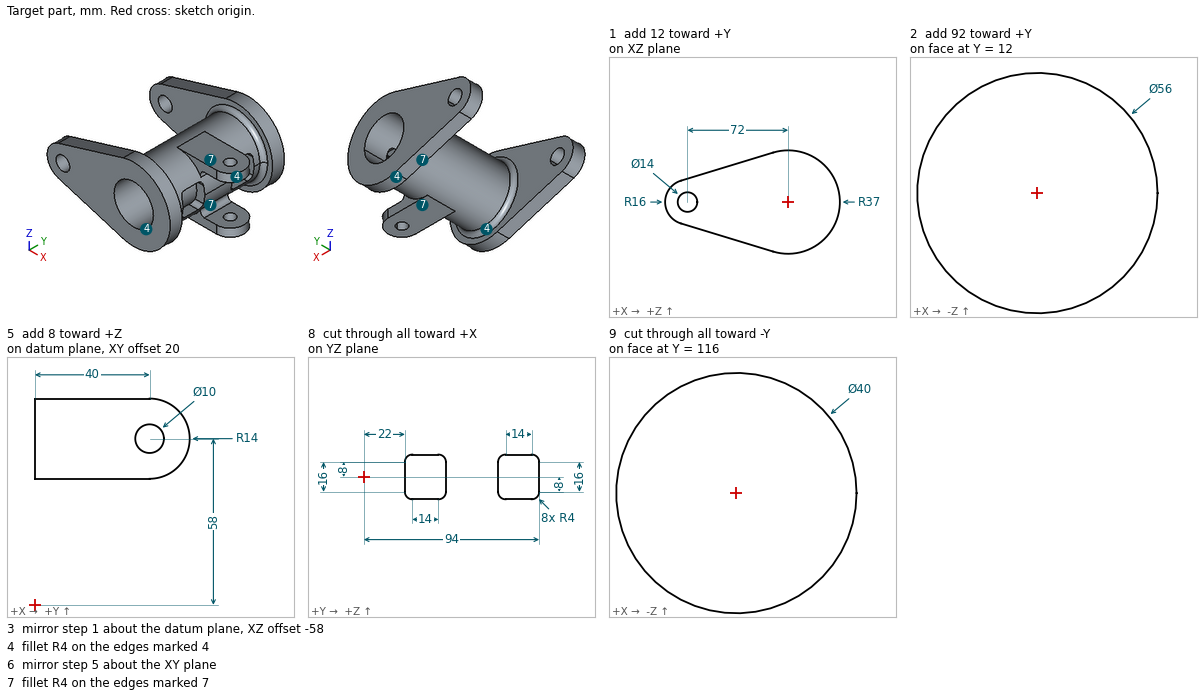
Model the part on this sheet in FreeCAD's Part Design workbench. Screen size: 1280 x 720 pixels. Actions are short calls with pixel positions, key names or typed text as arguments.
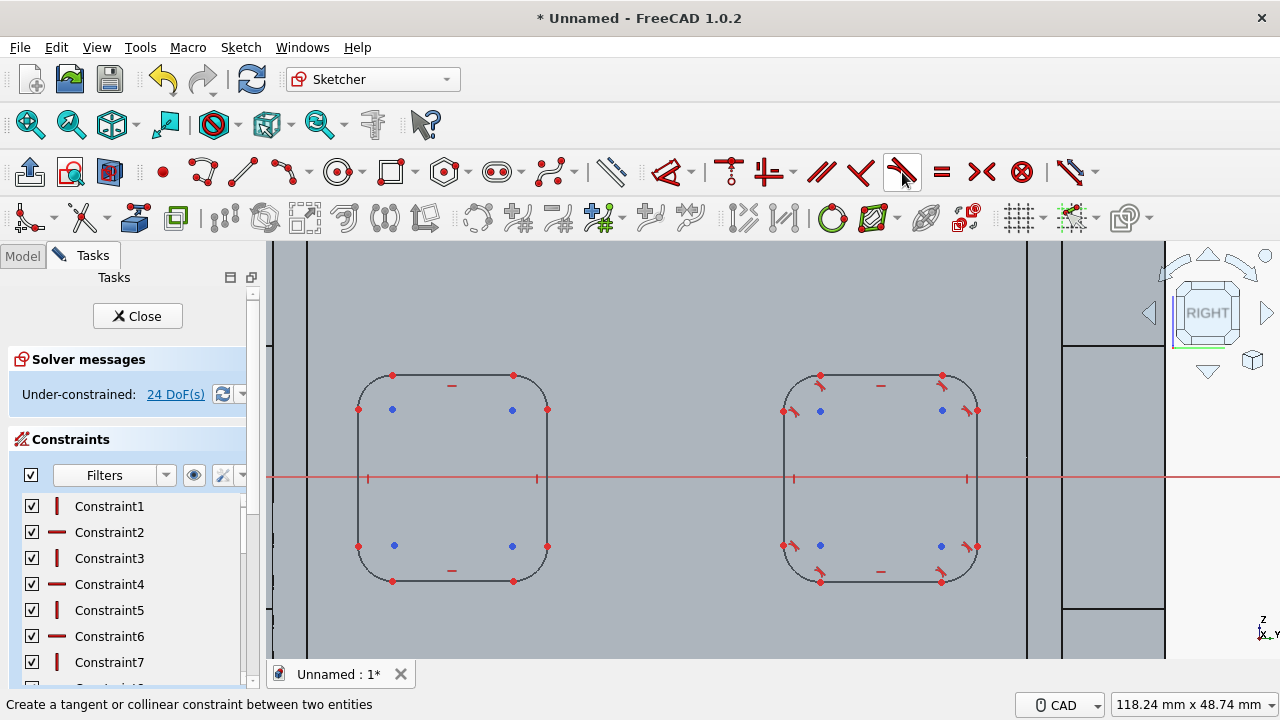
click(358, 451)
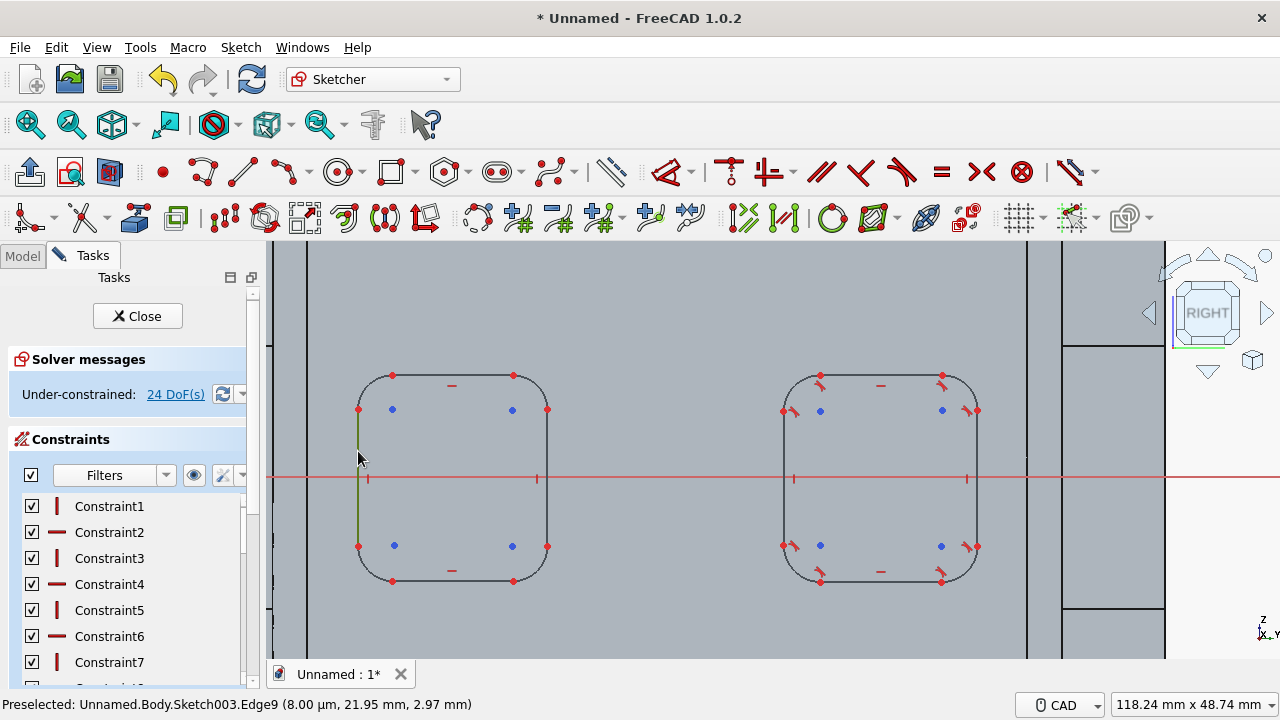
click(362, 562)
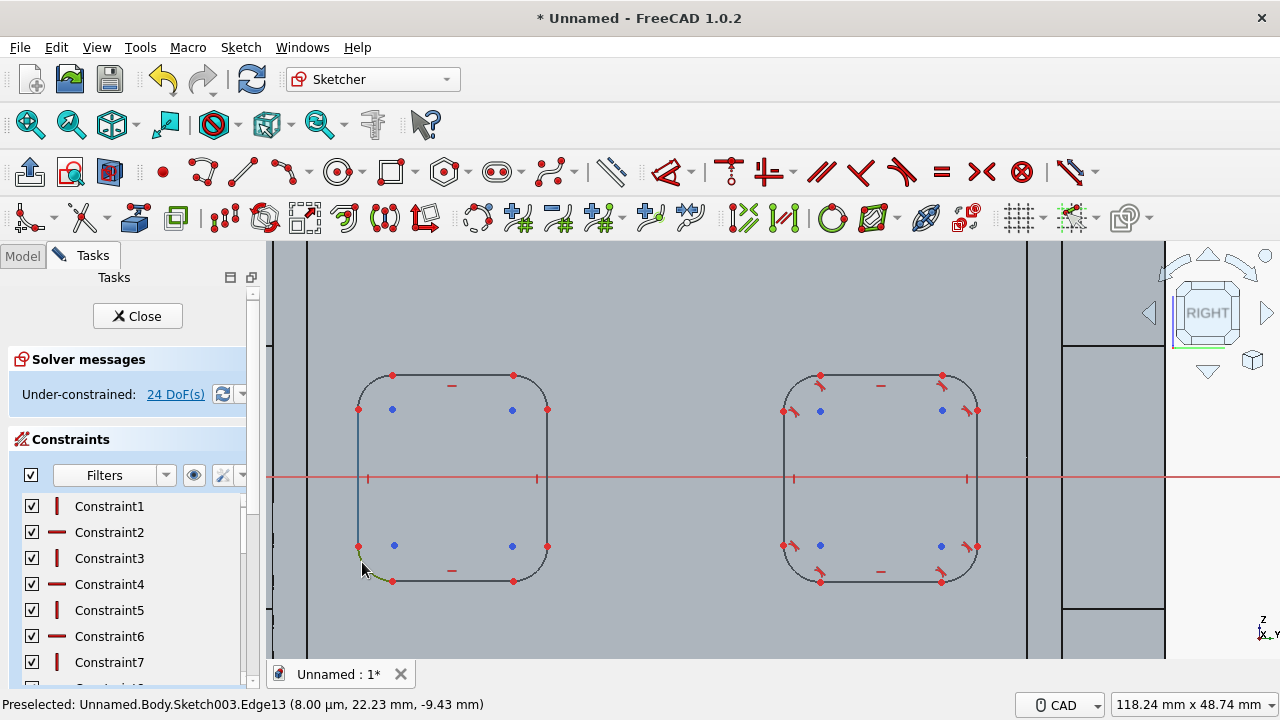
key(t)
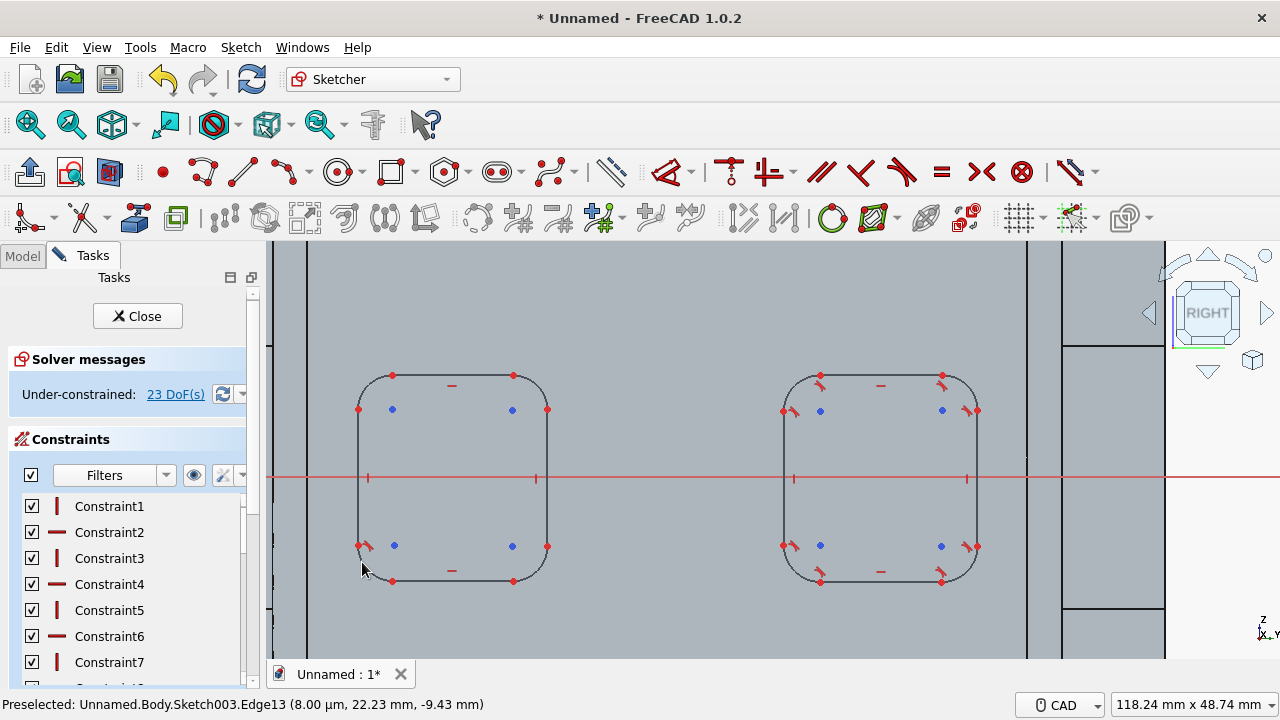
click(358, 450)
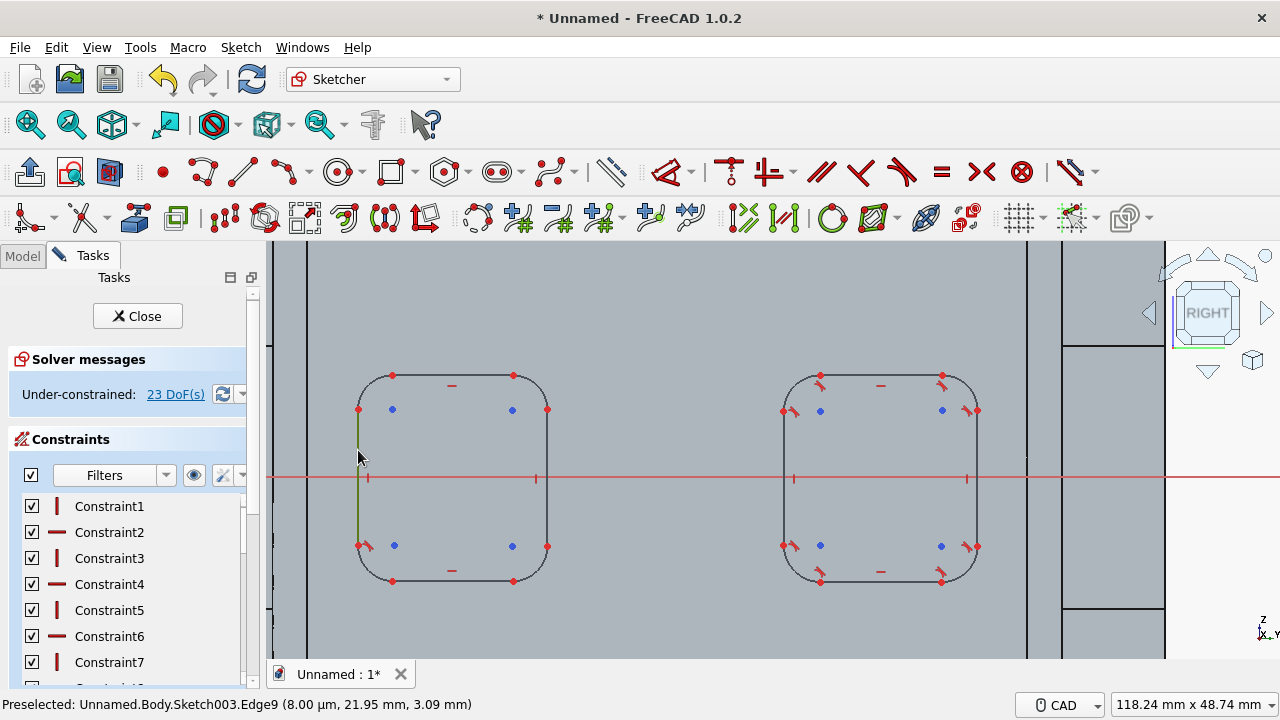
click(377, 379)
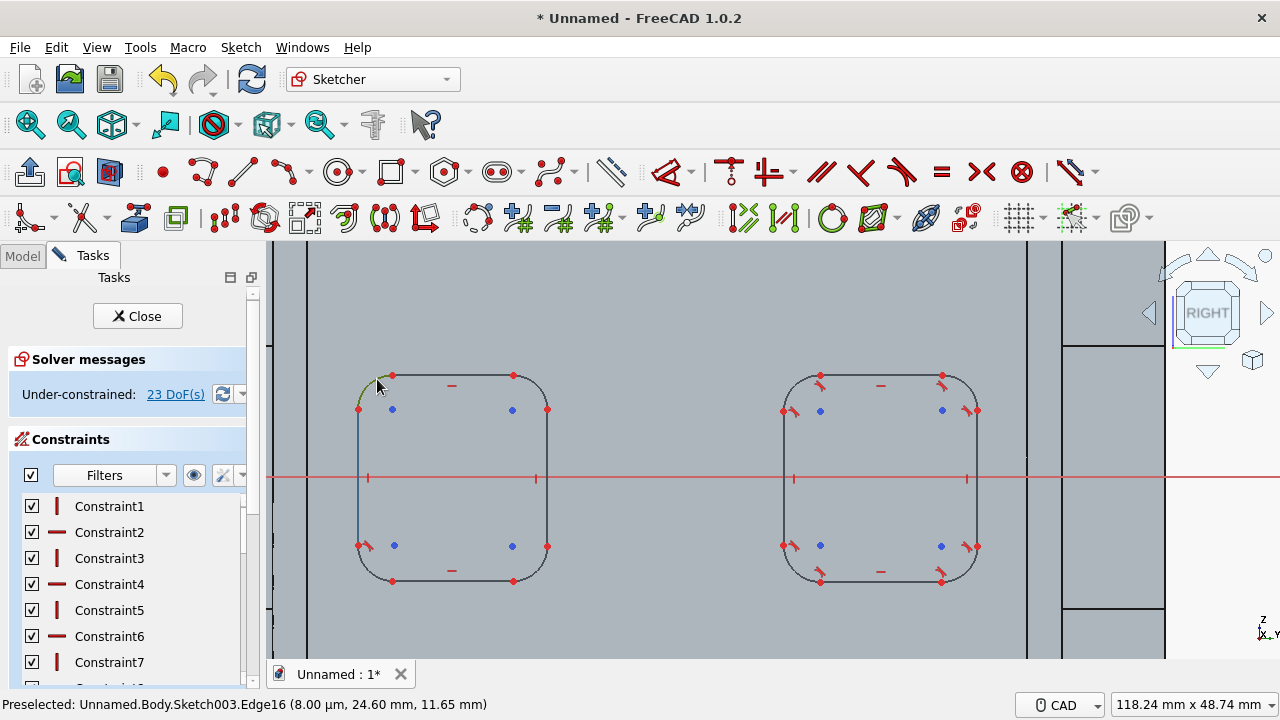
click(902, 172)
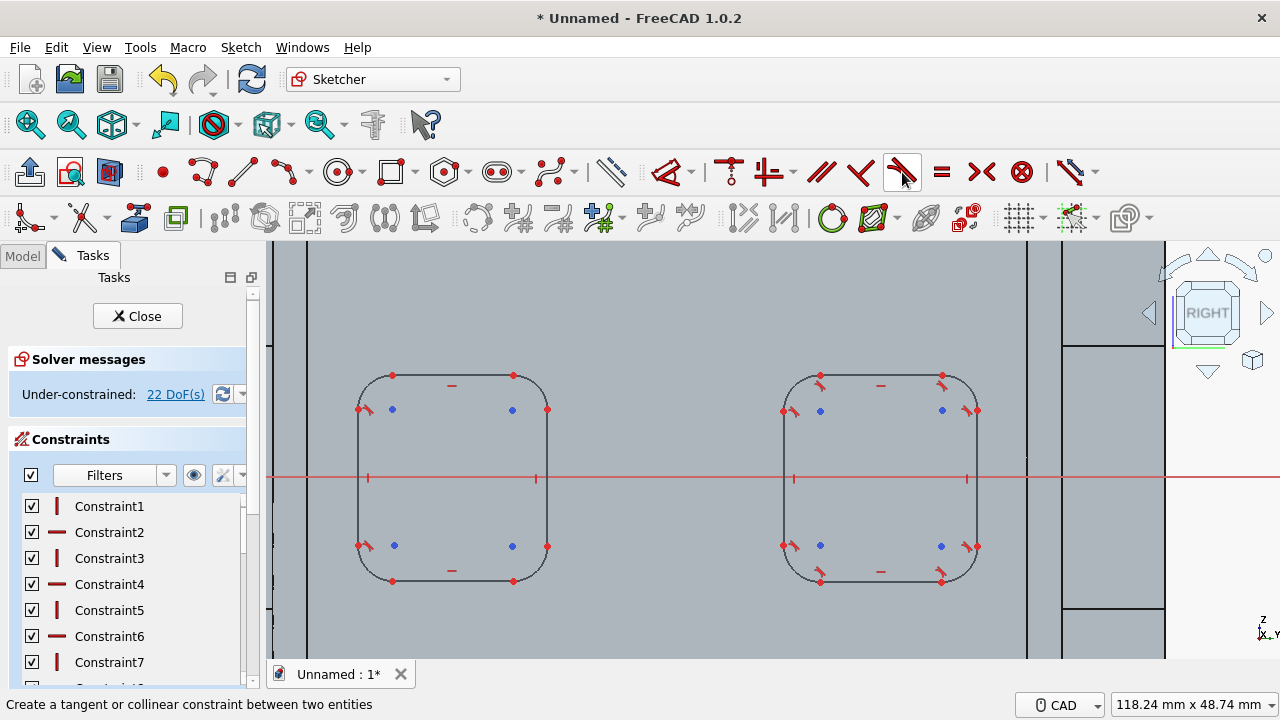
click(429, 581)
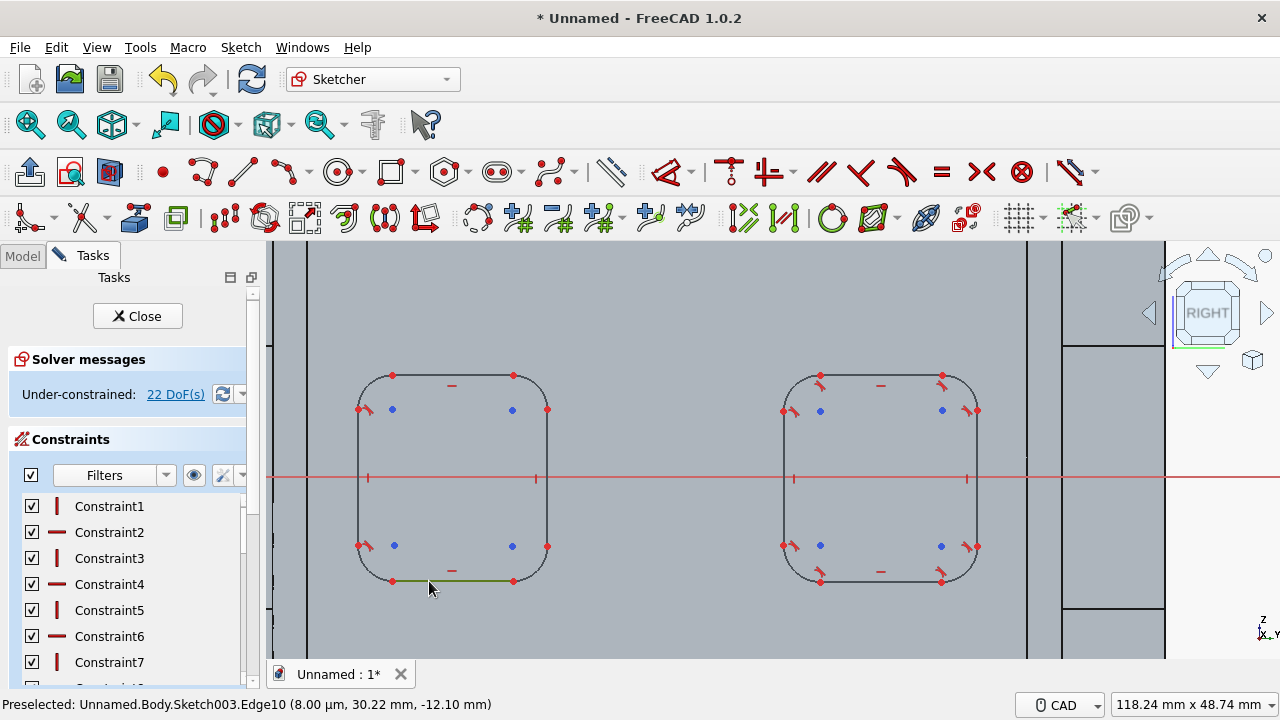
click(362, 561)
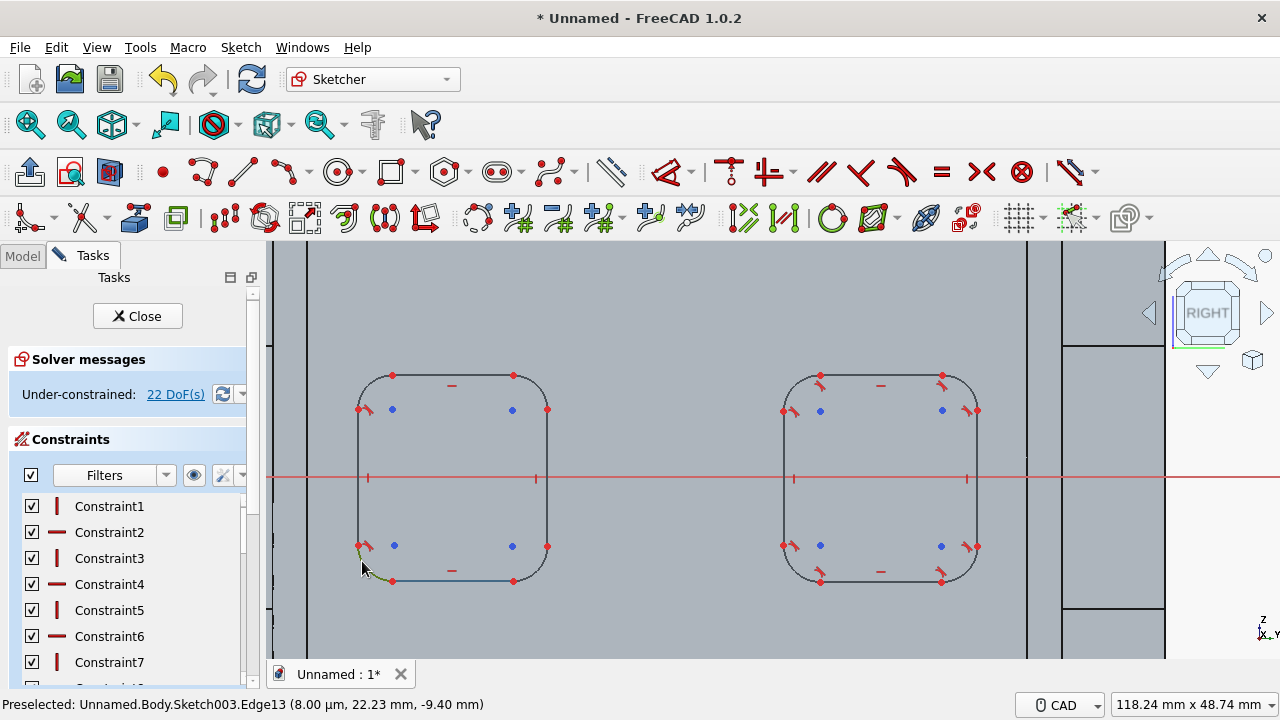
click(902, 172)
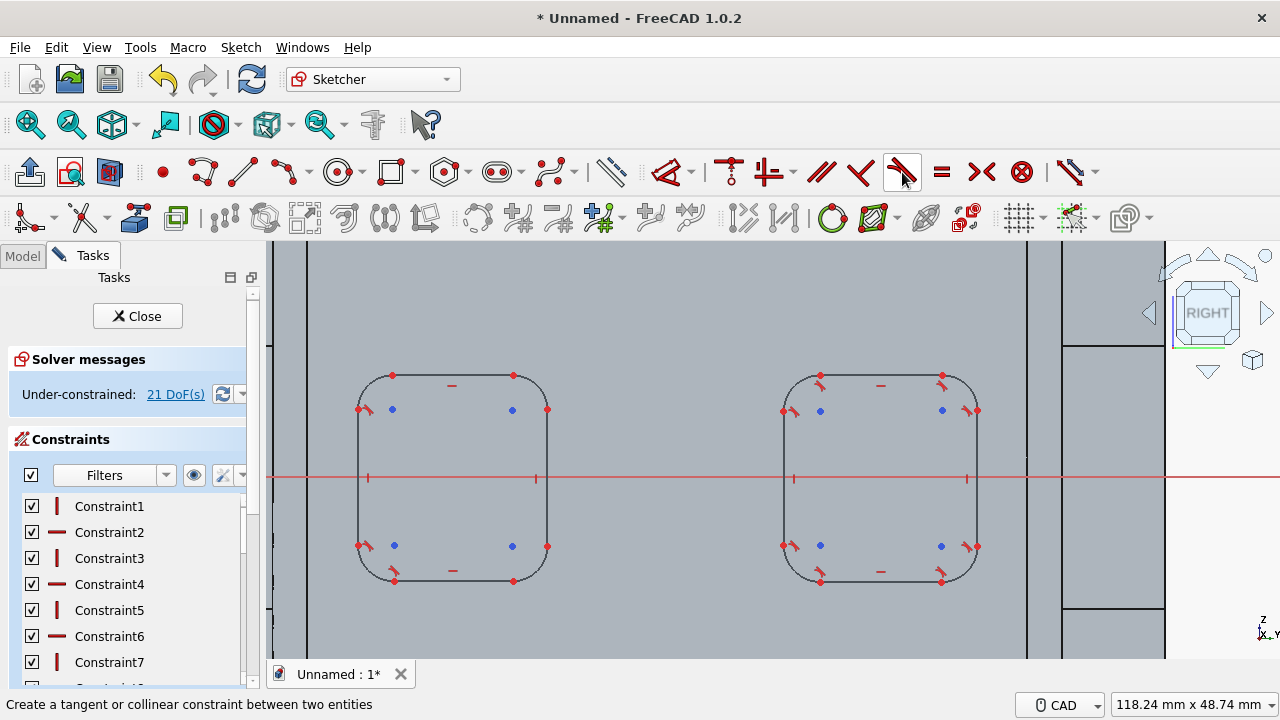
click(430, 581)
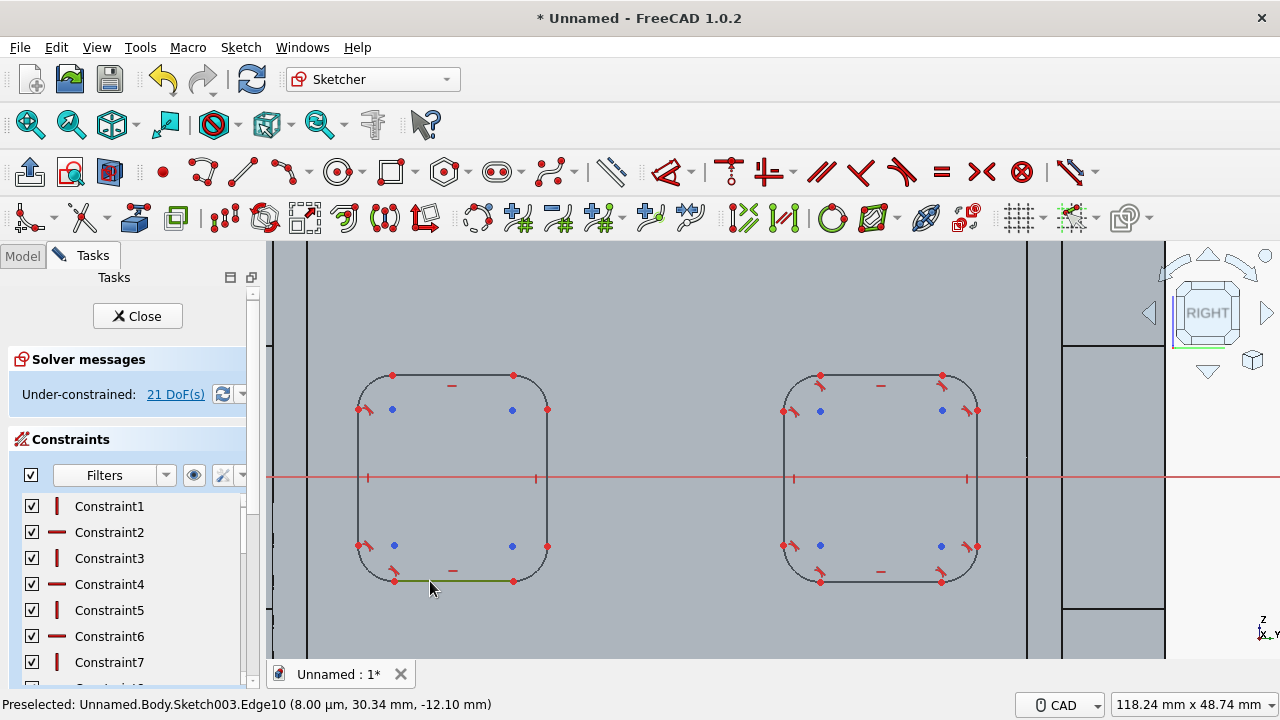
click(529, 577)